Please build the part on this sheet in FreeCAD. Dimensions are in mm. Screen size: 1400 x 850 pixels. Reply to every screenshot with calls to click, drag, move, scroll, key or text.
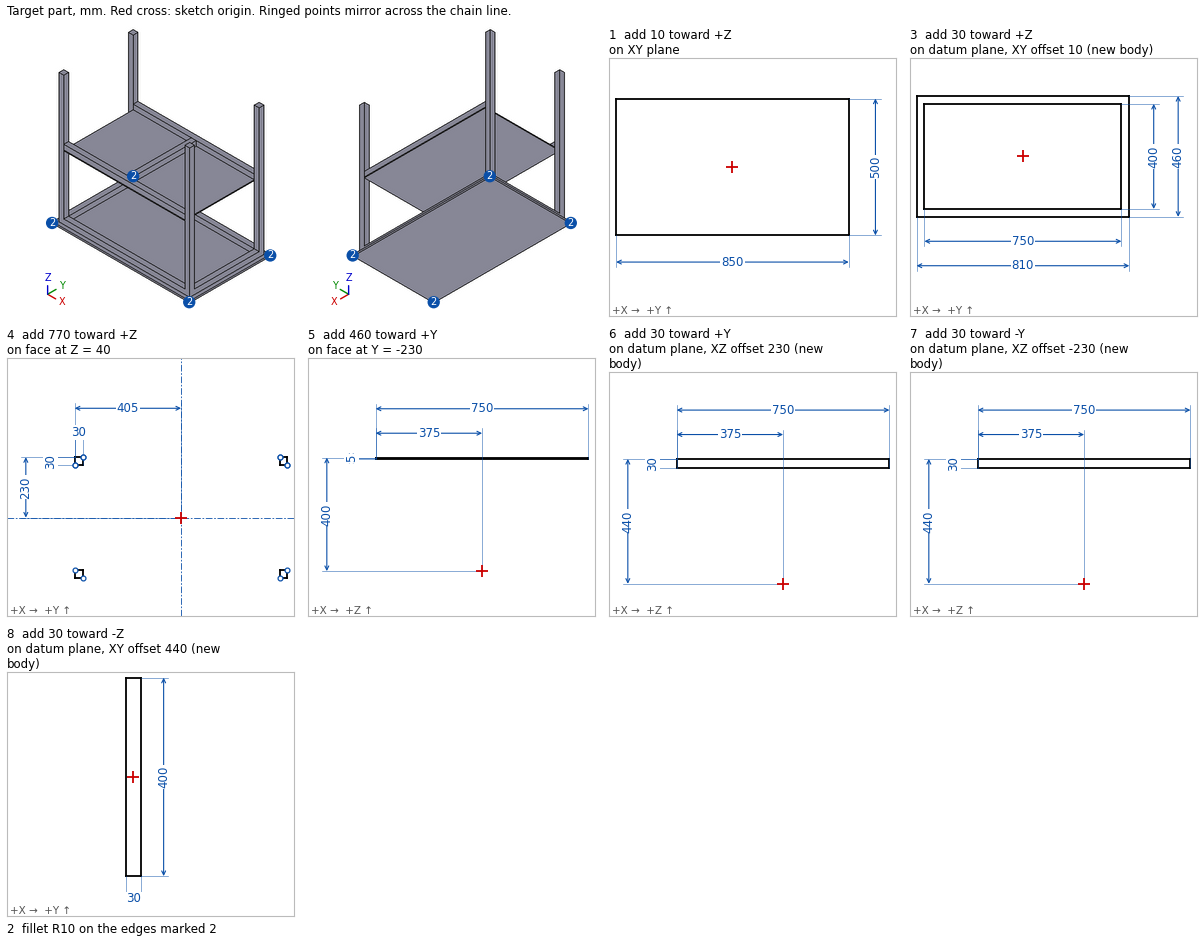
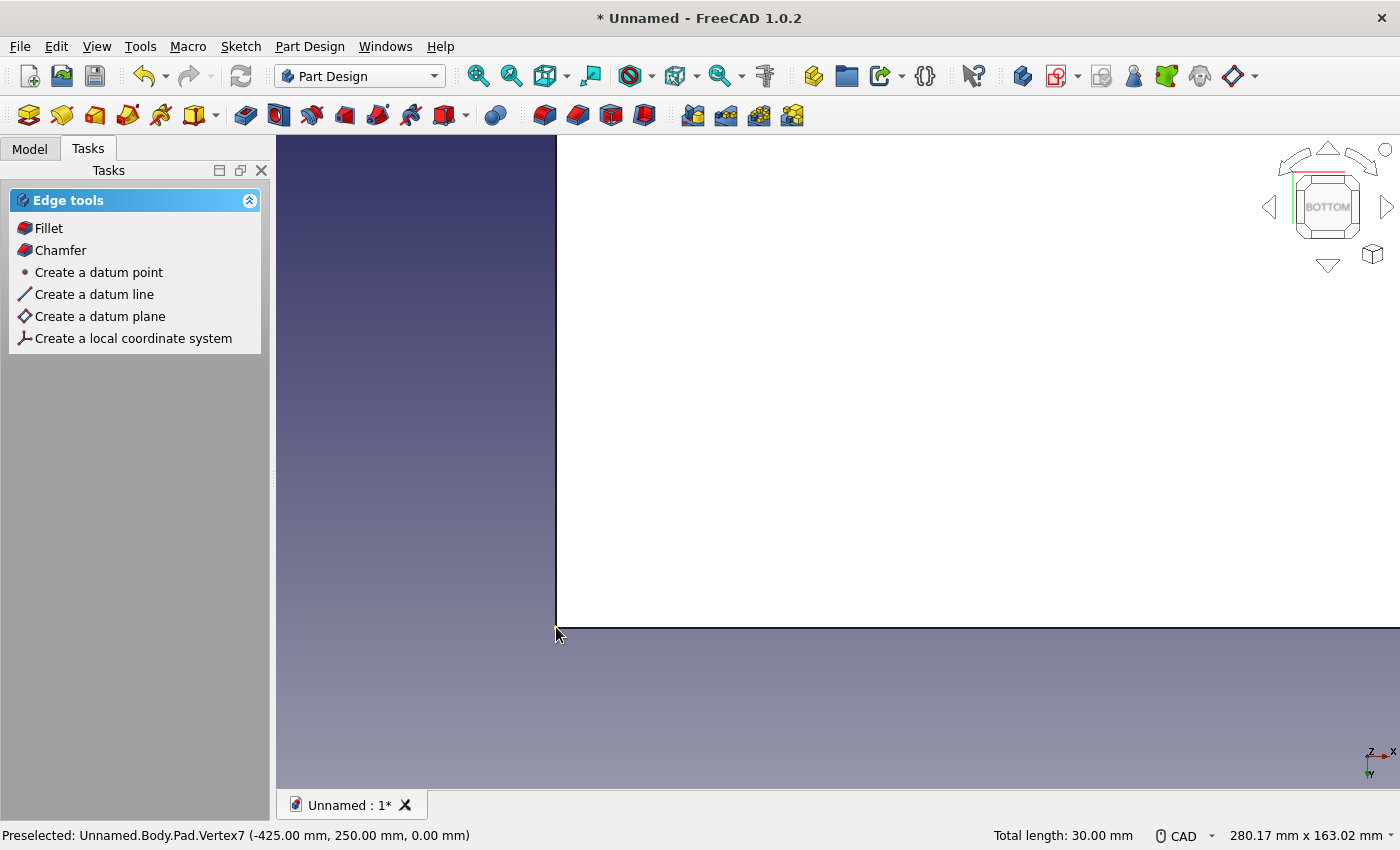
key(v)
key(f)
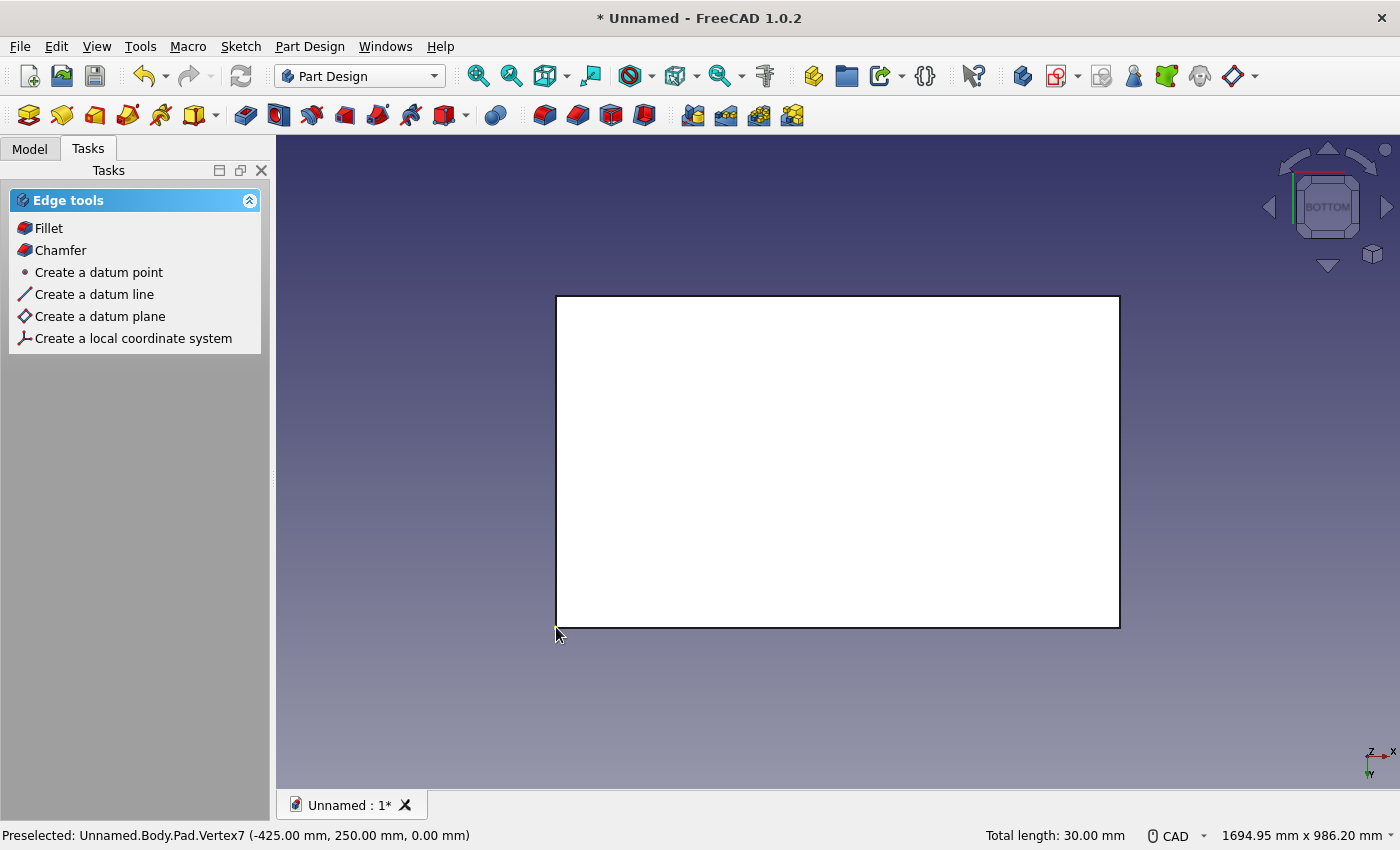
key(4)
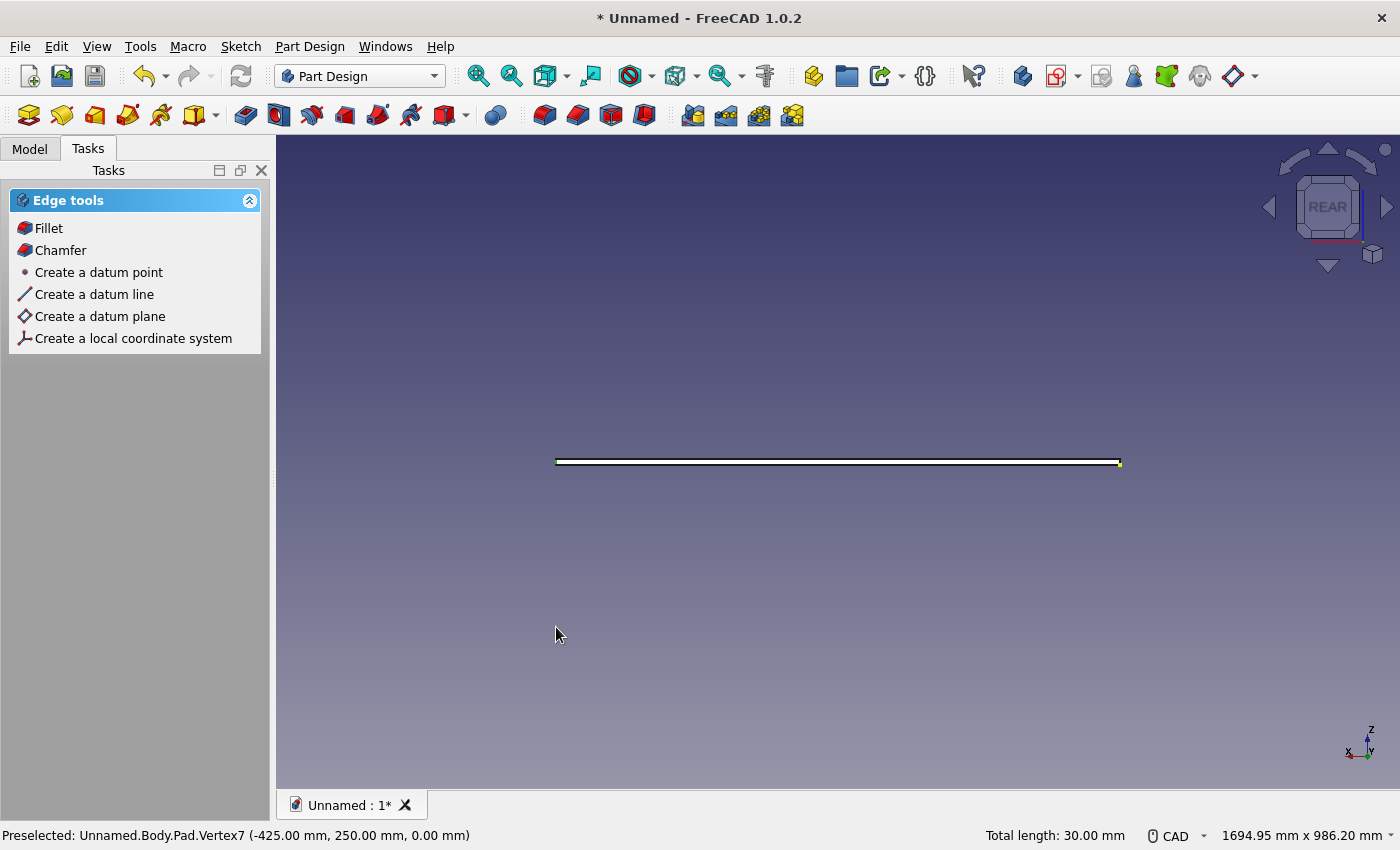
scroll(1120, 461, up, 9)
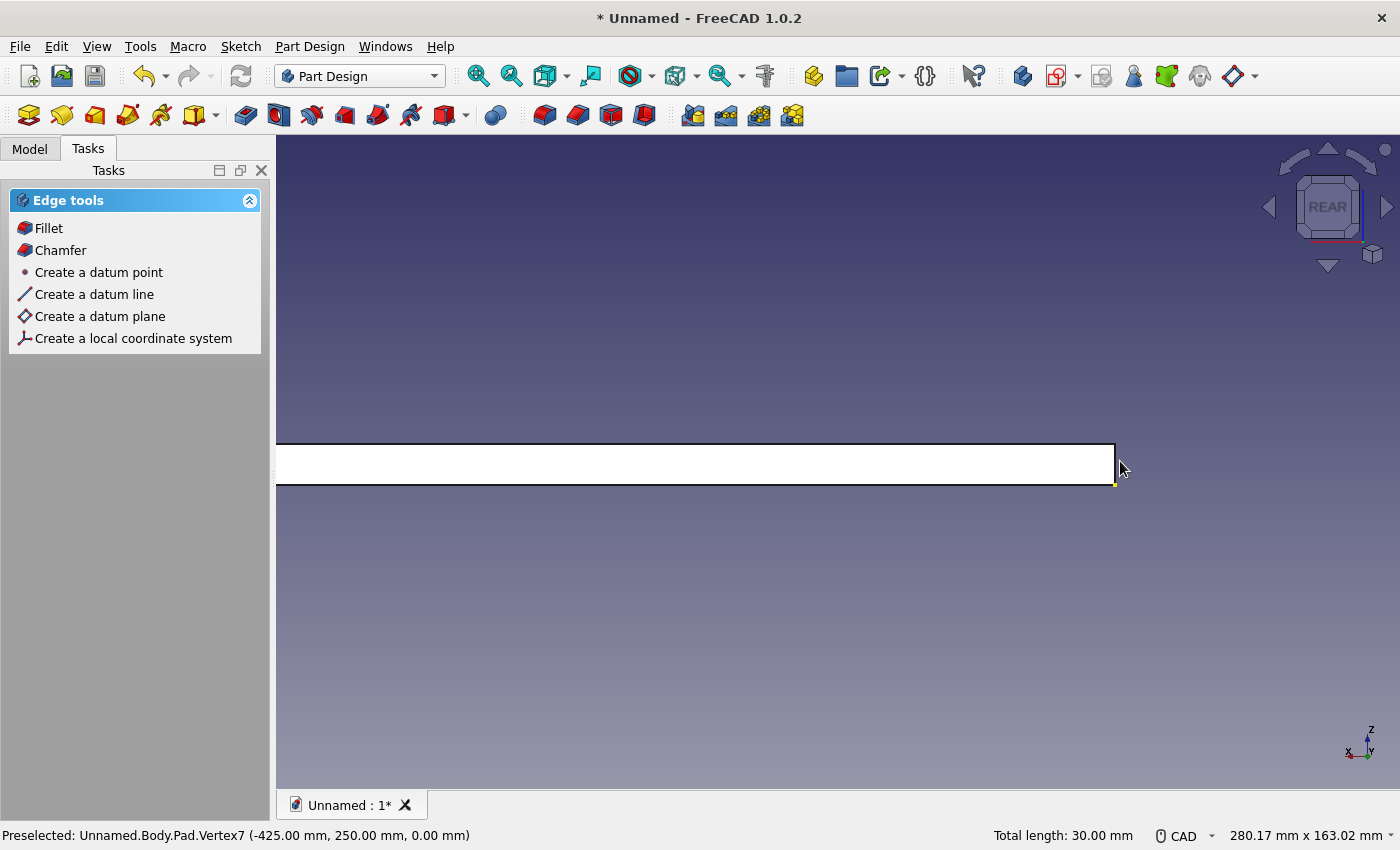
click(1115, 464, ctrl)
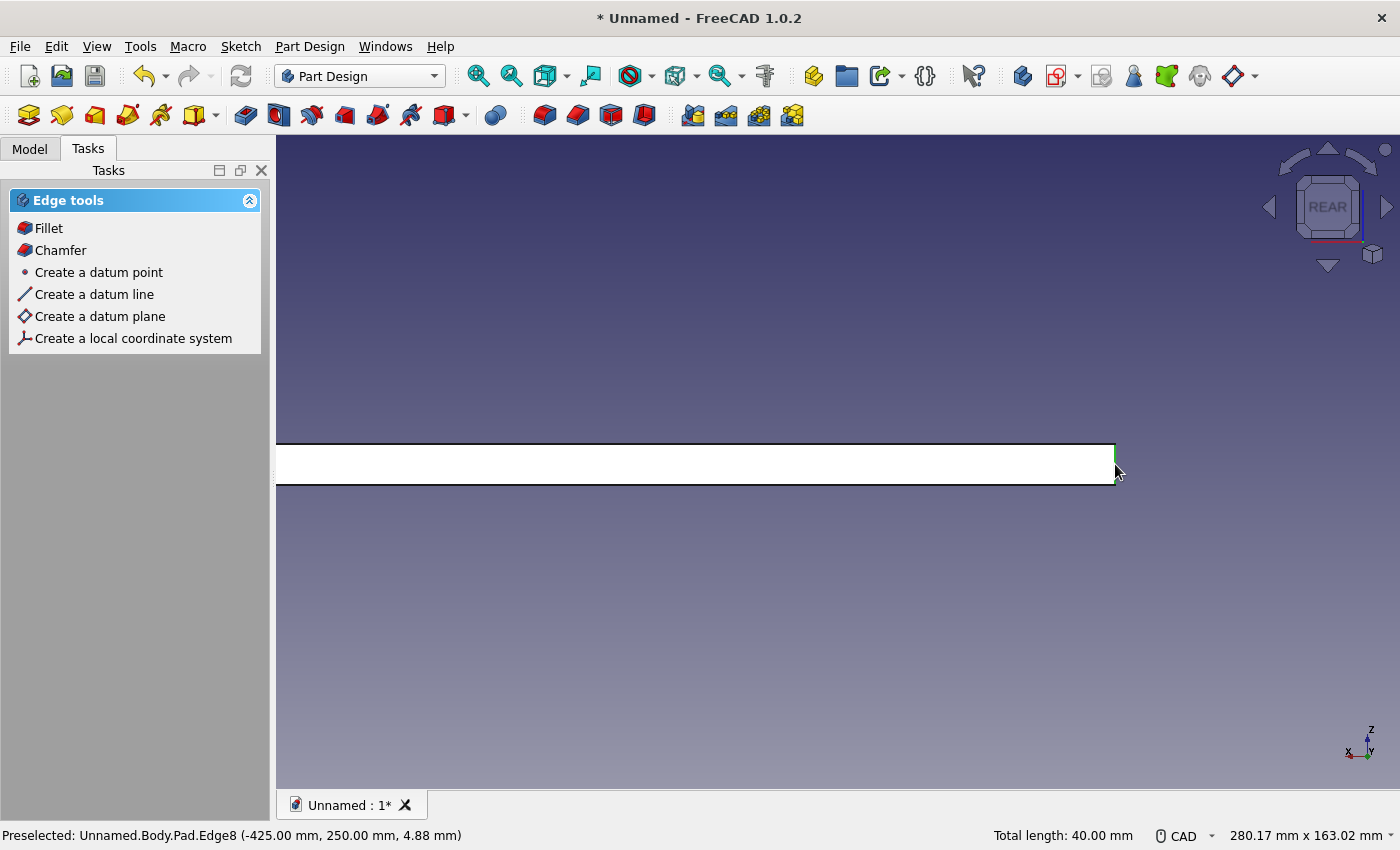
click(545, 116)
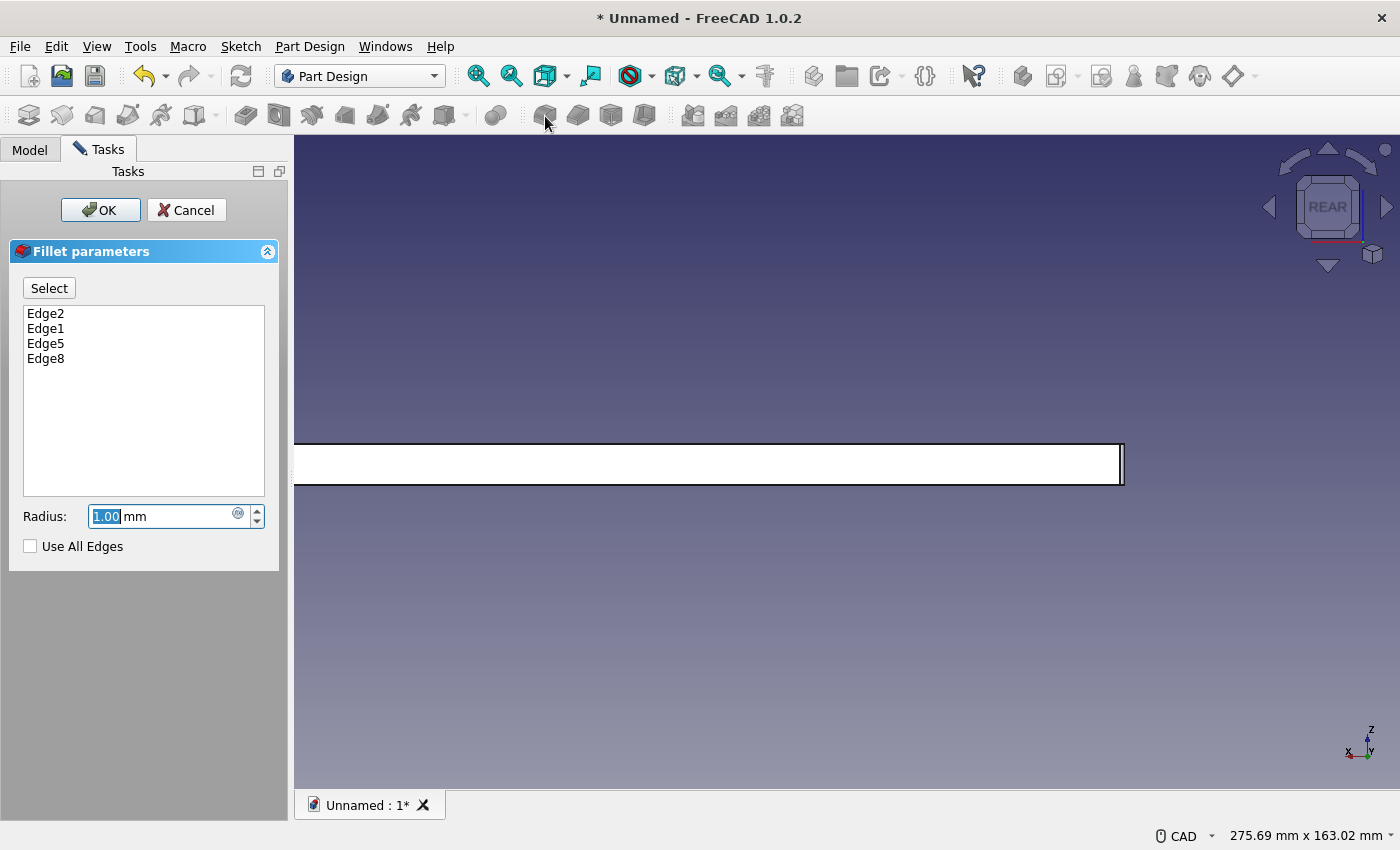
text(10)
key(Tab)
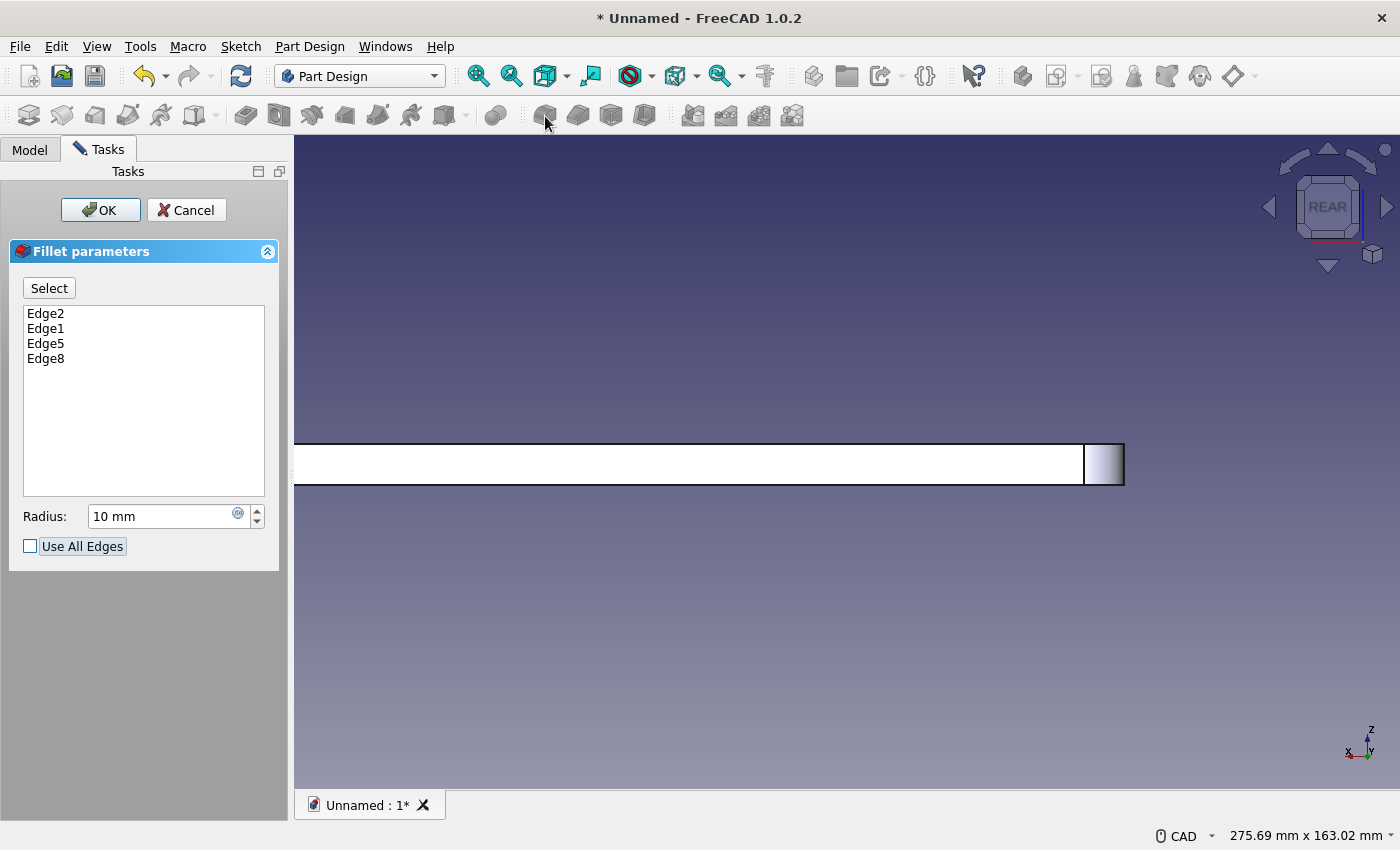
click(101, 210)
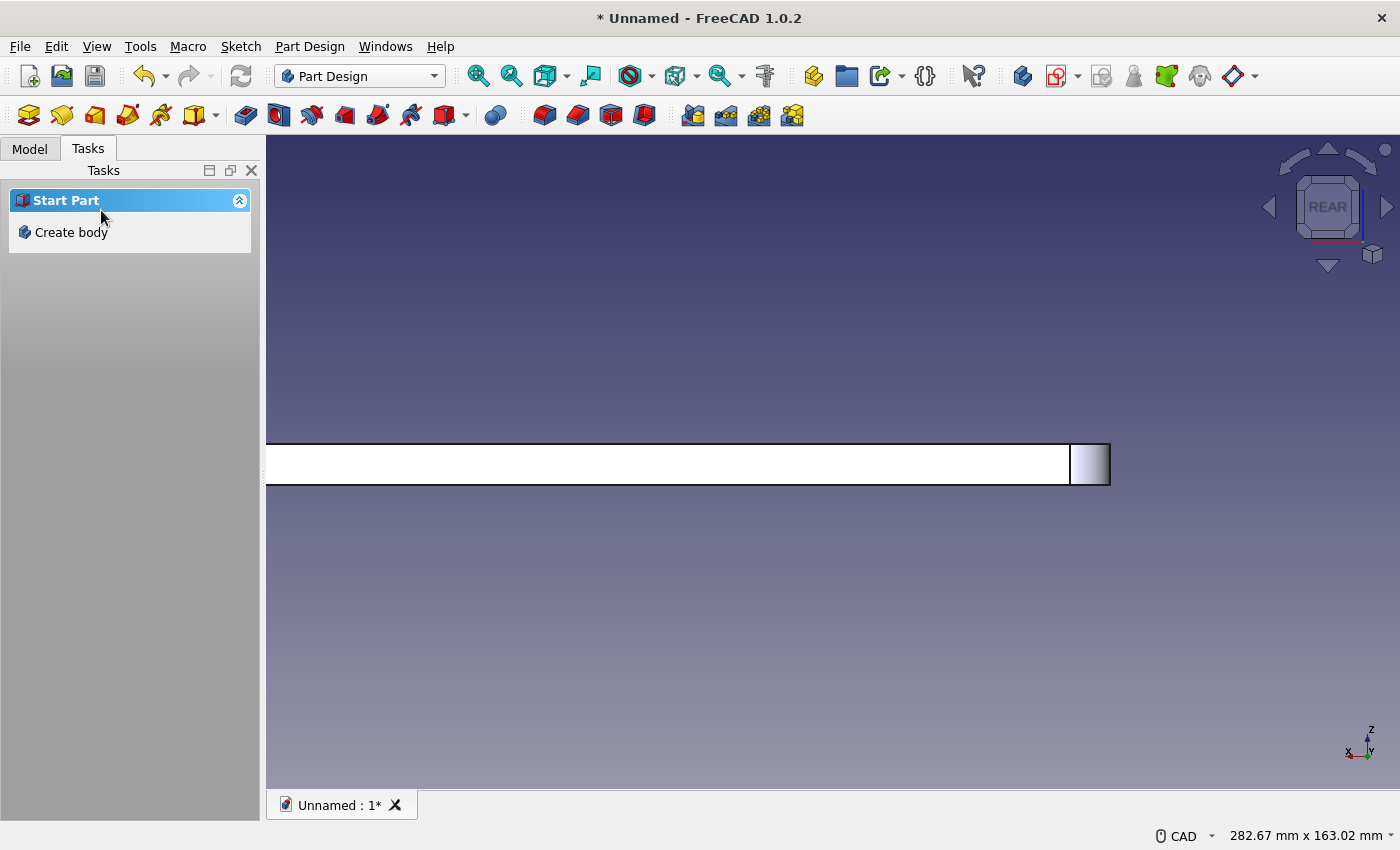
click(479, 76)